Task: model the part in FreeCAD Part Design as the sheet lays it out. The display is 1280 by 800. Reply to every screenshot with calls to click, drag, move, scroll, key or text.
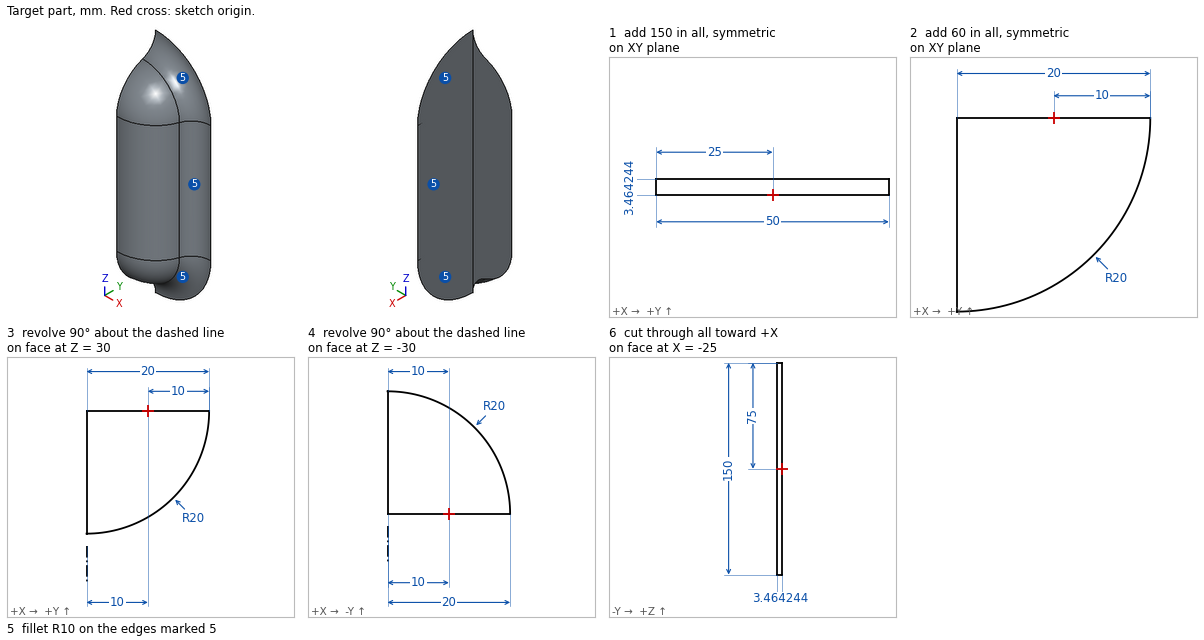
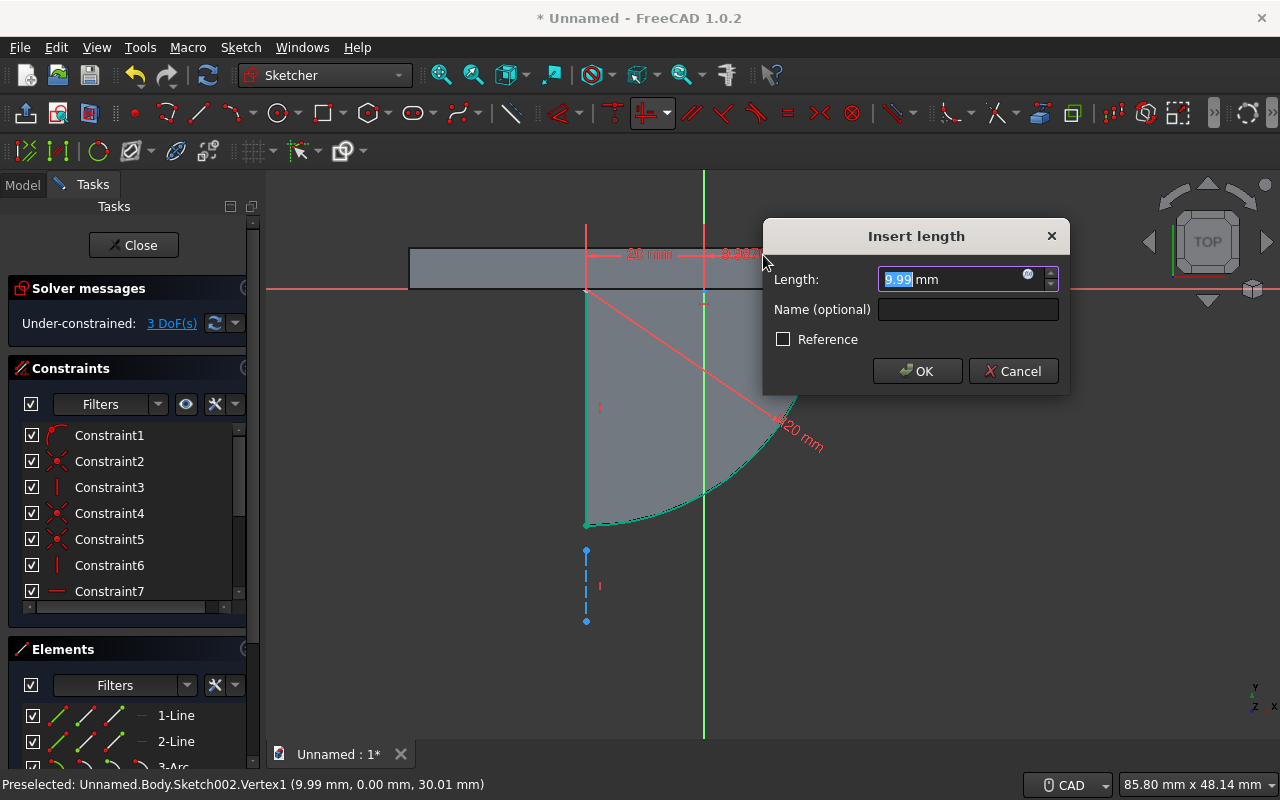
text(10)
key(Return)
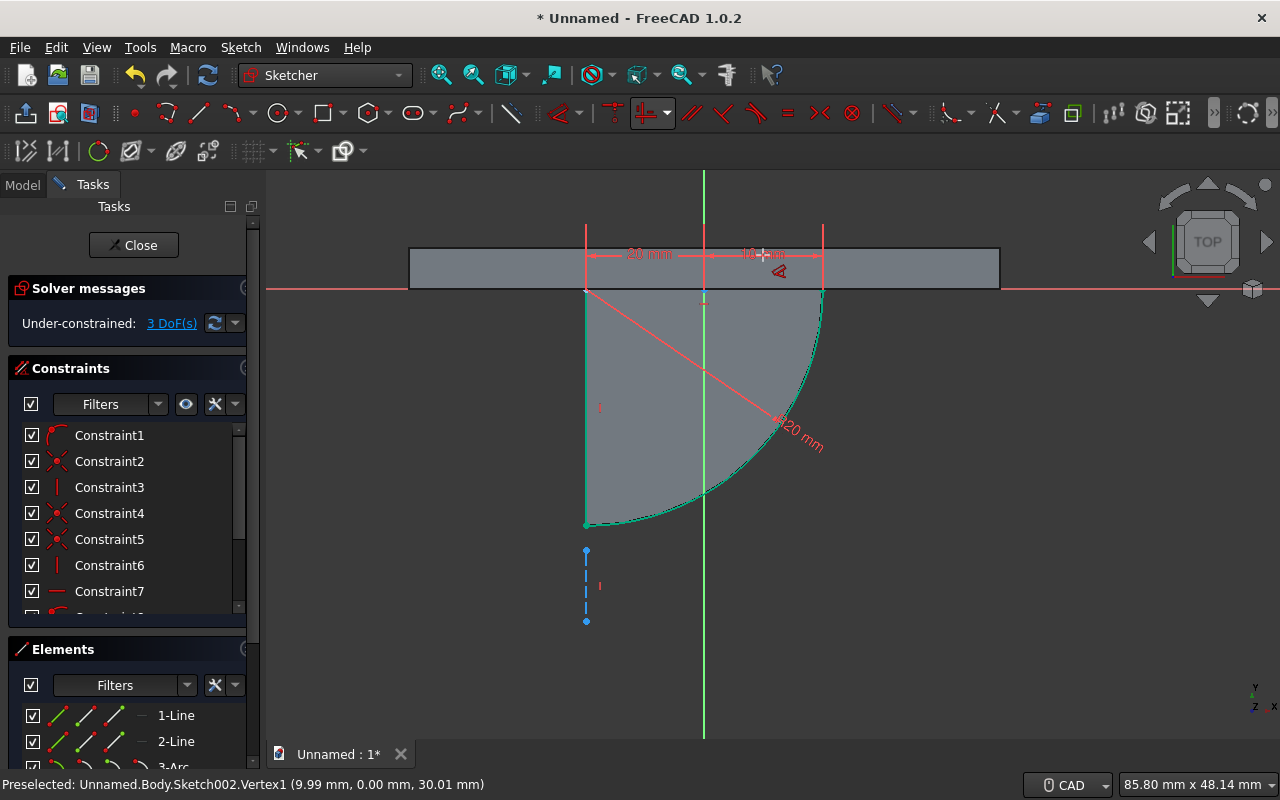
click(586, 550)
click(645, 584)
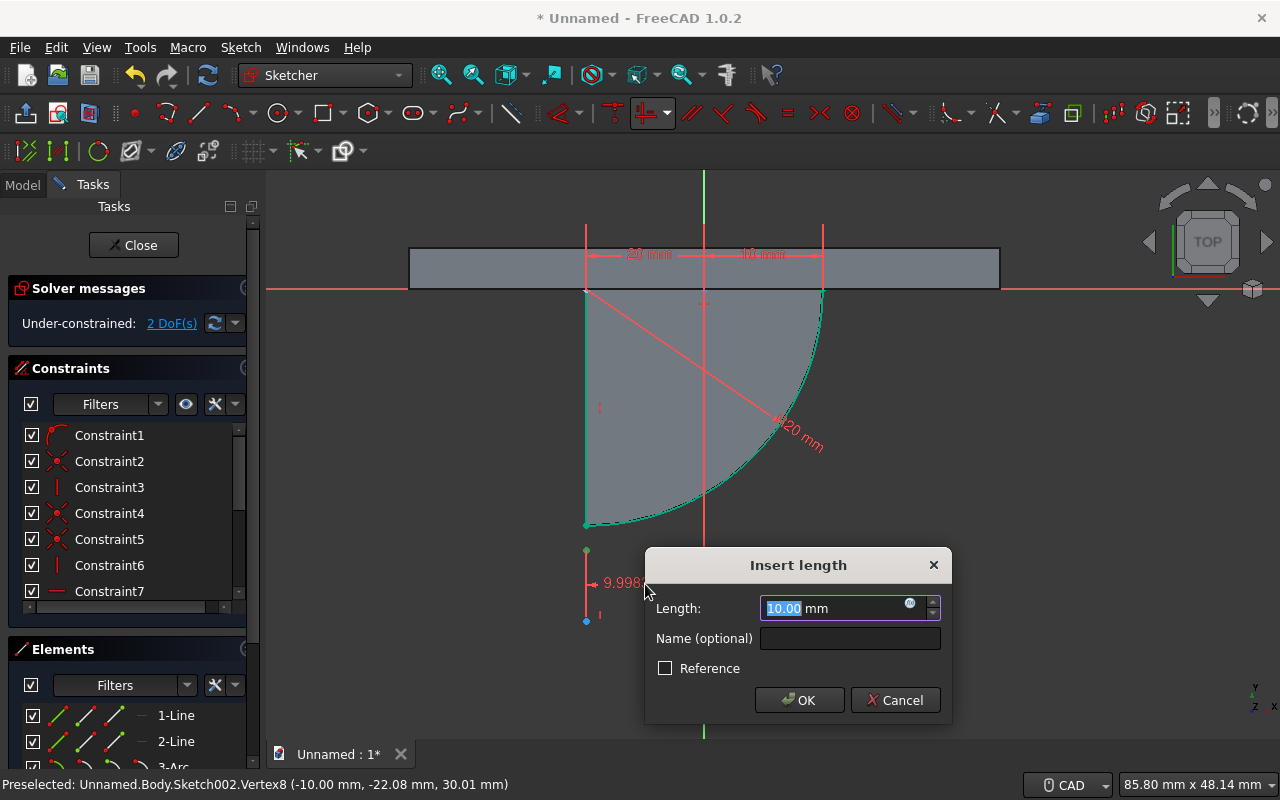
text(10)
key(Return)
key(Escape)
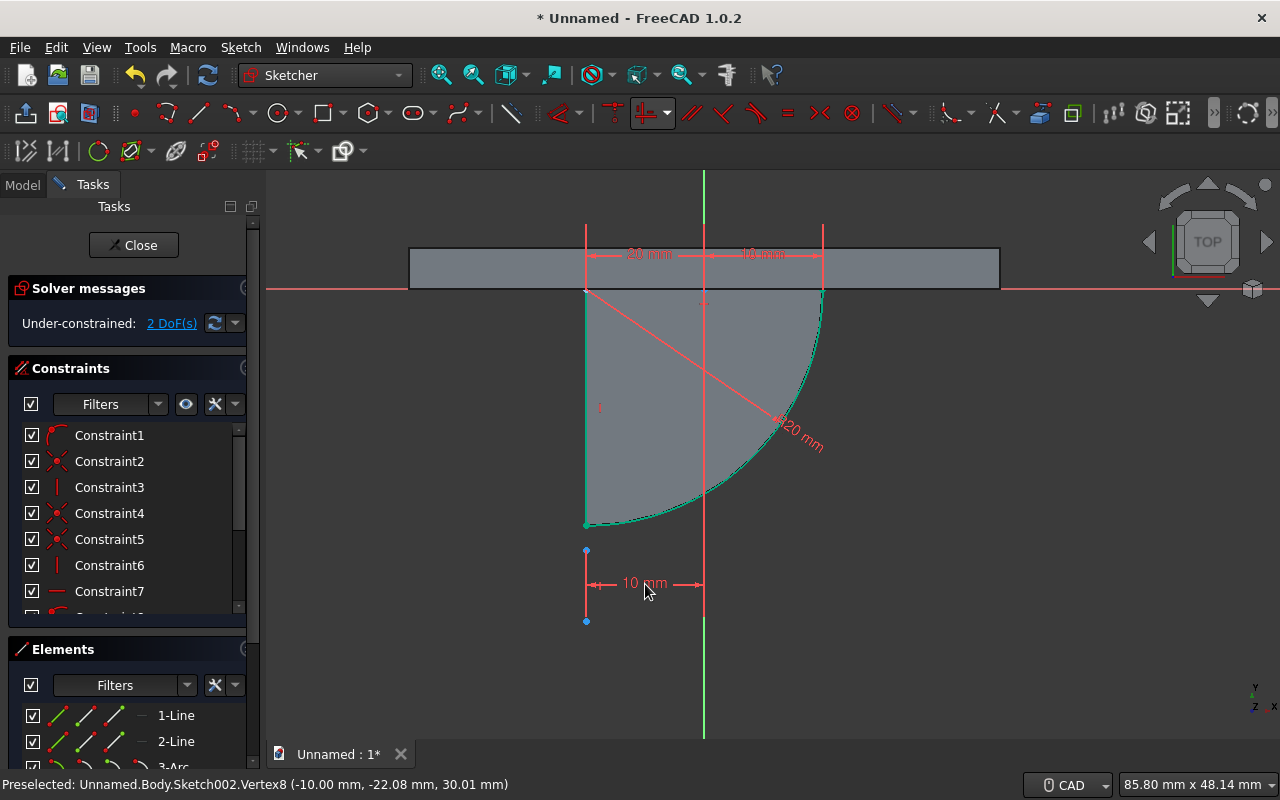
click(134, 245)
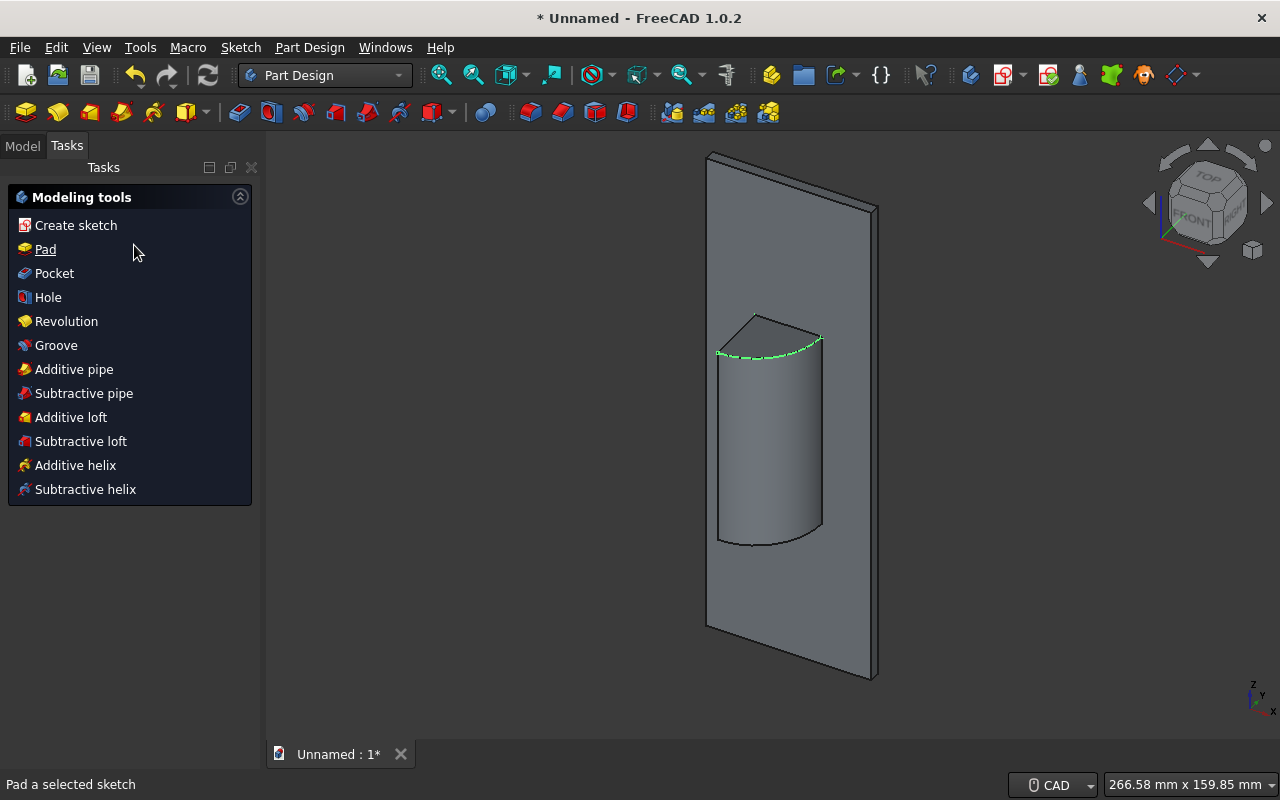
click(58, 112)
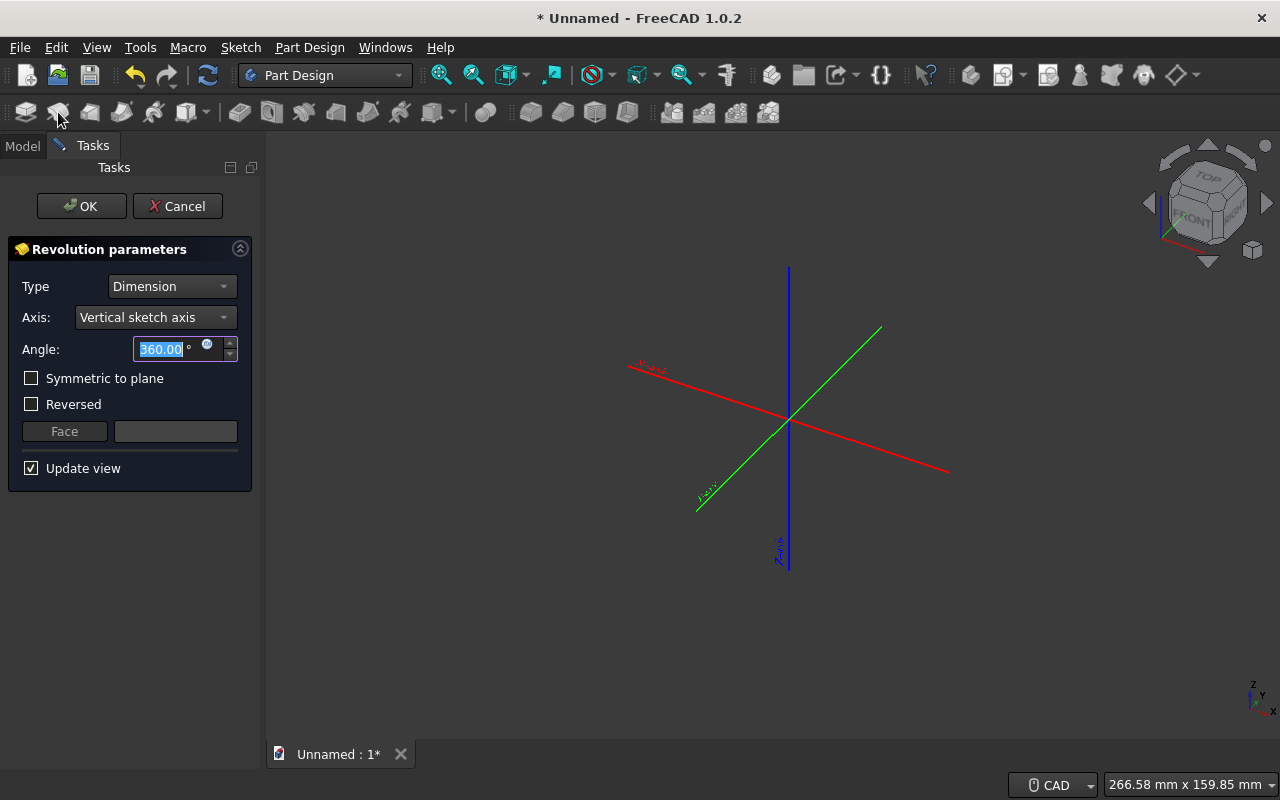
click(156, 318)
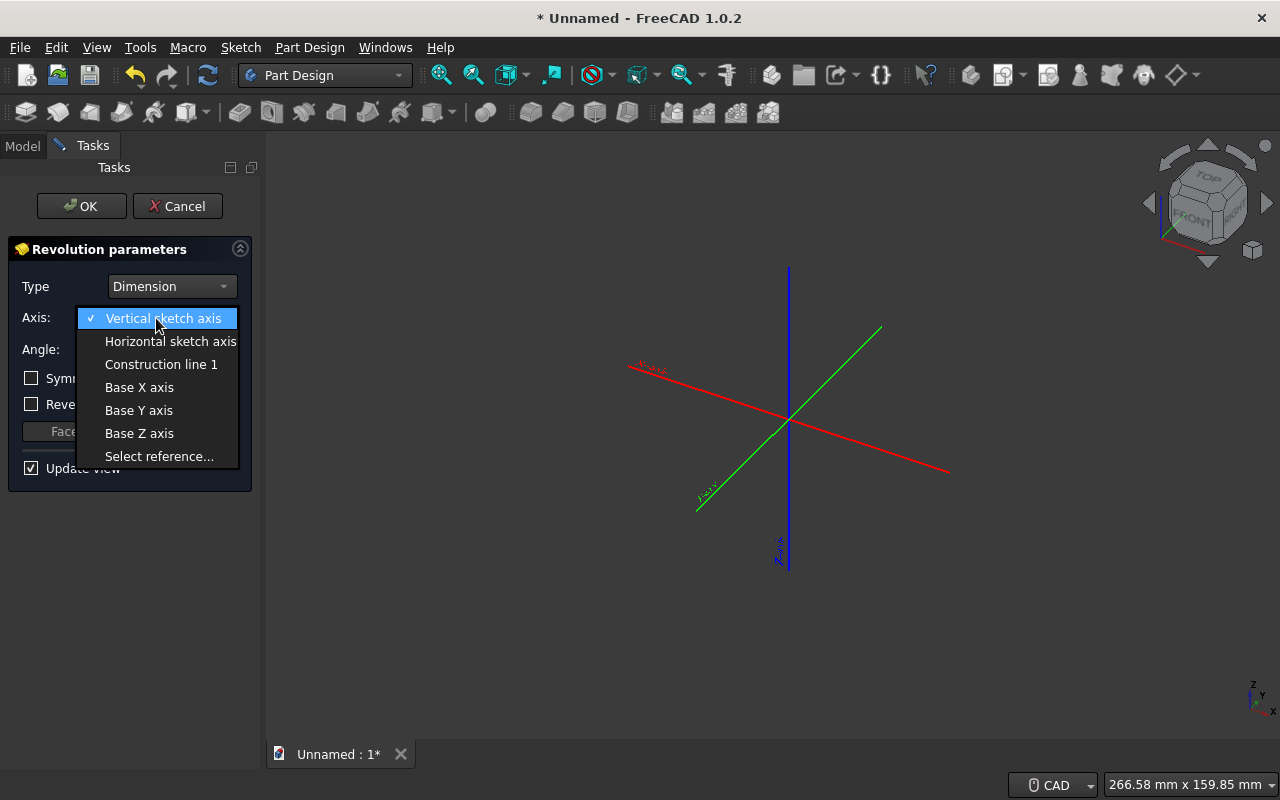
click(156, 364)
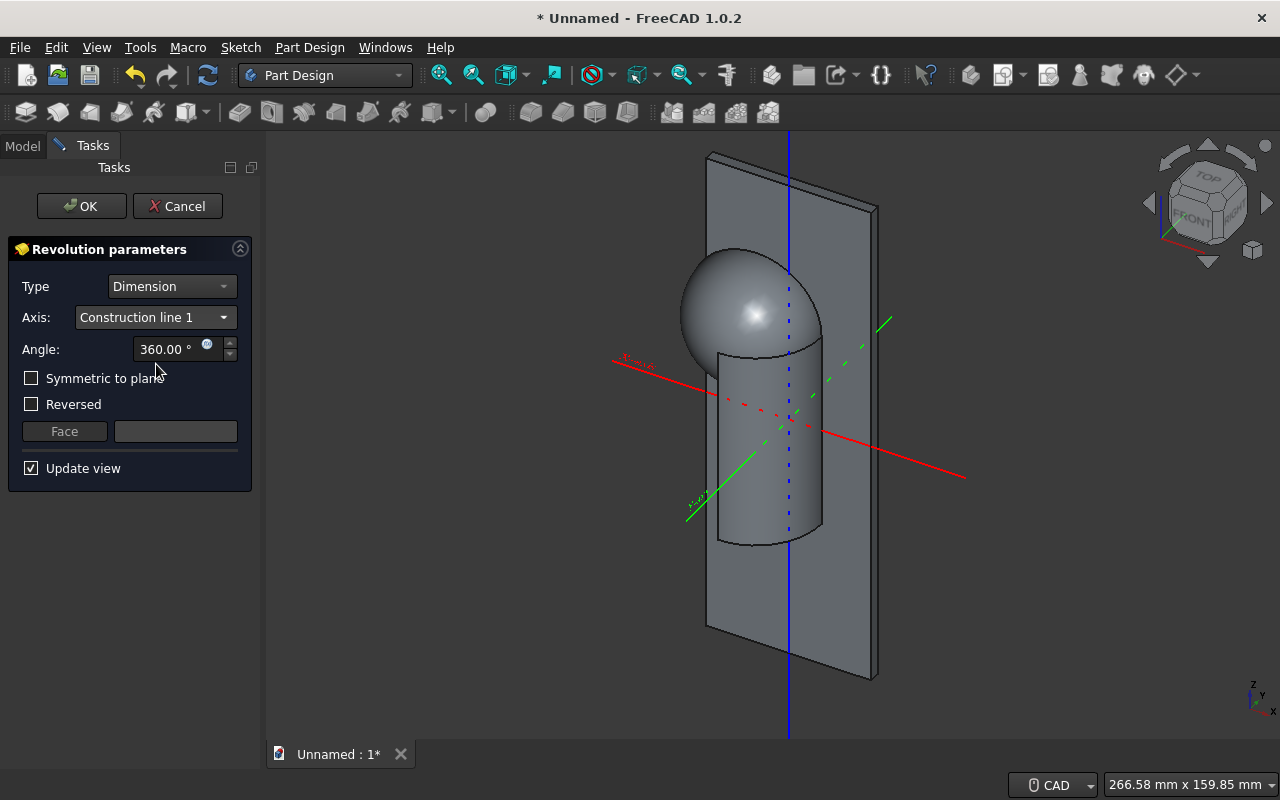
triple_click(178, 349)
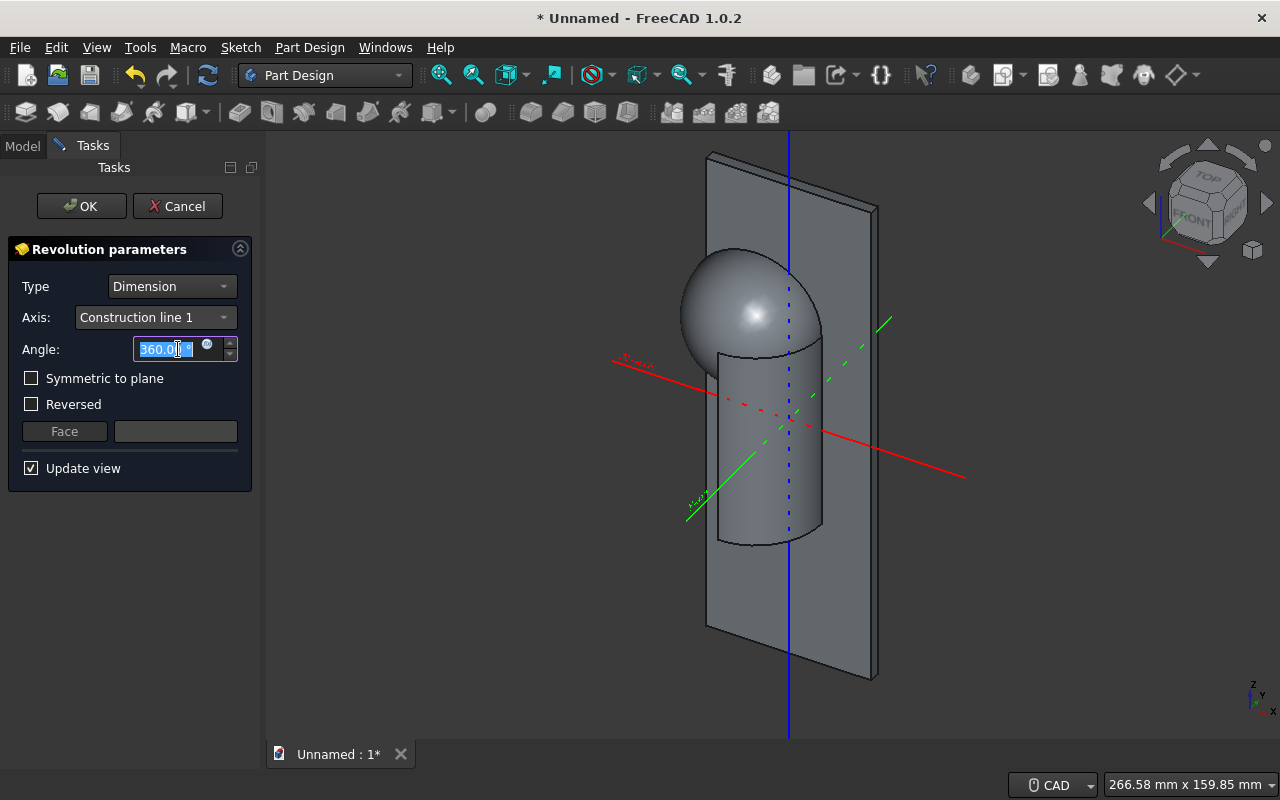
text(90)
key(Tab)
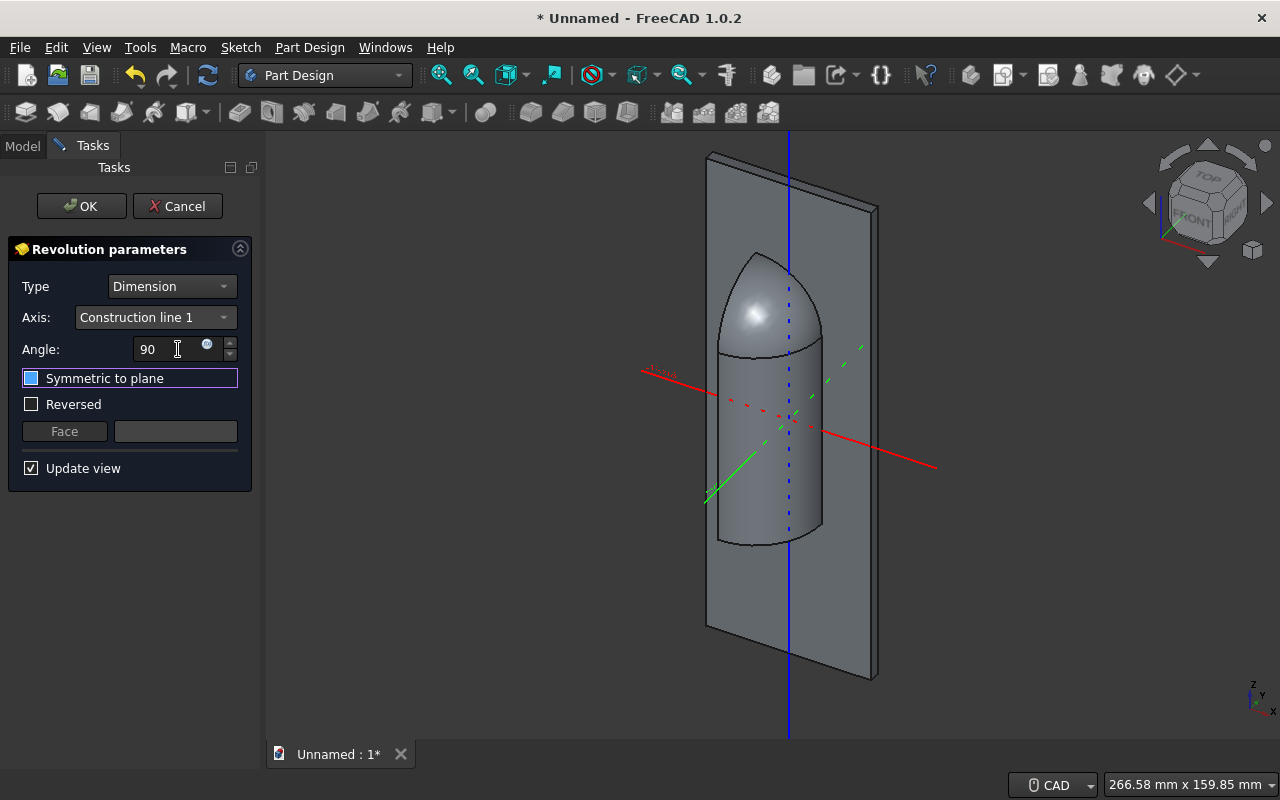
click(82, 206)